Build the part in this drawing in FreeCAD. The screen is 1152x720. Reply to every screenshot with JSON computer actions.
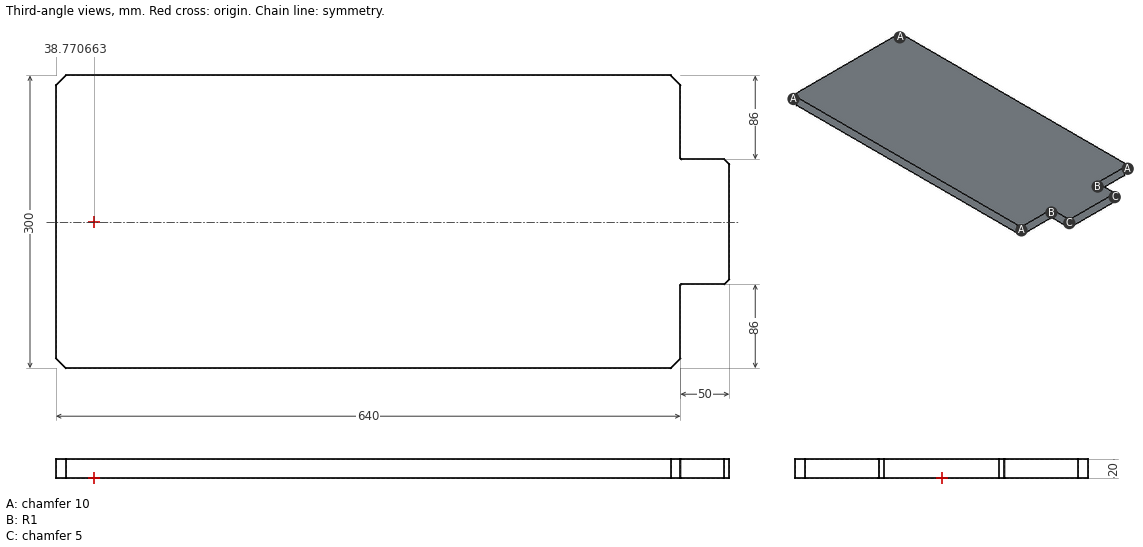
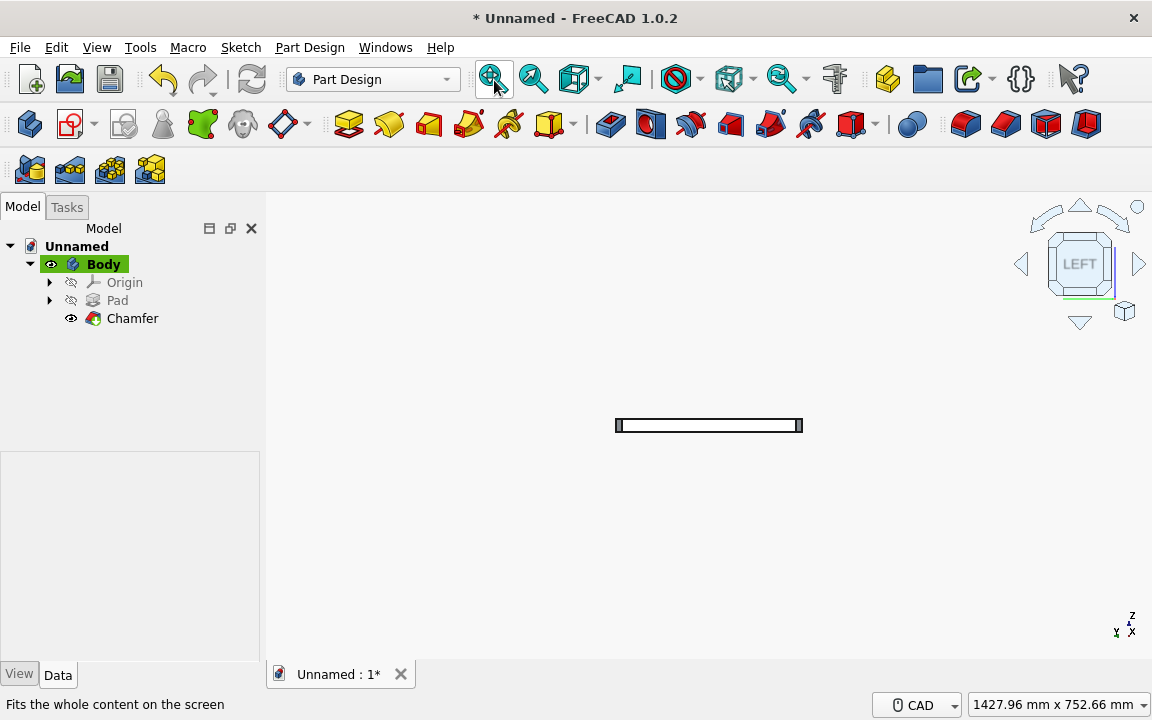
{"action": "left_click", "coordinate": [494, 80]}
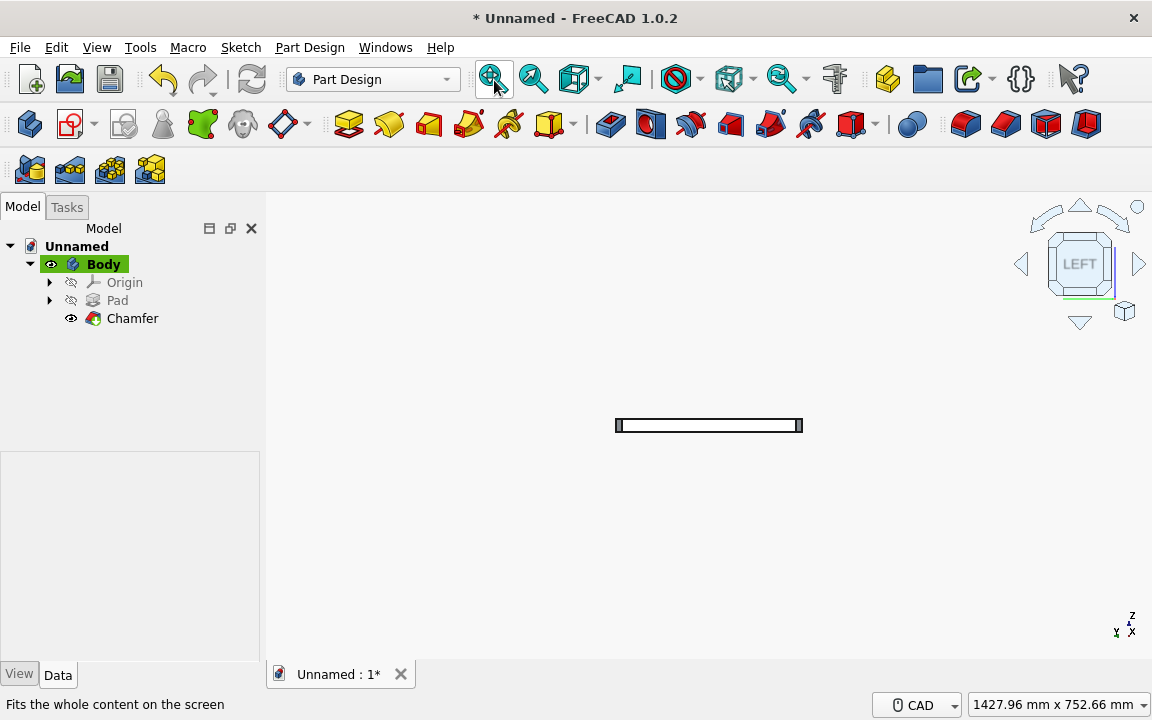
{"action": "scroll", "coordinate": [669, 424], "scroll_direction": "up", "scroll_amount": 6}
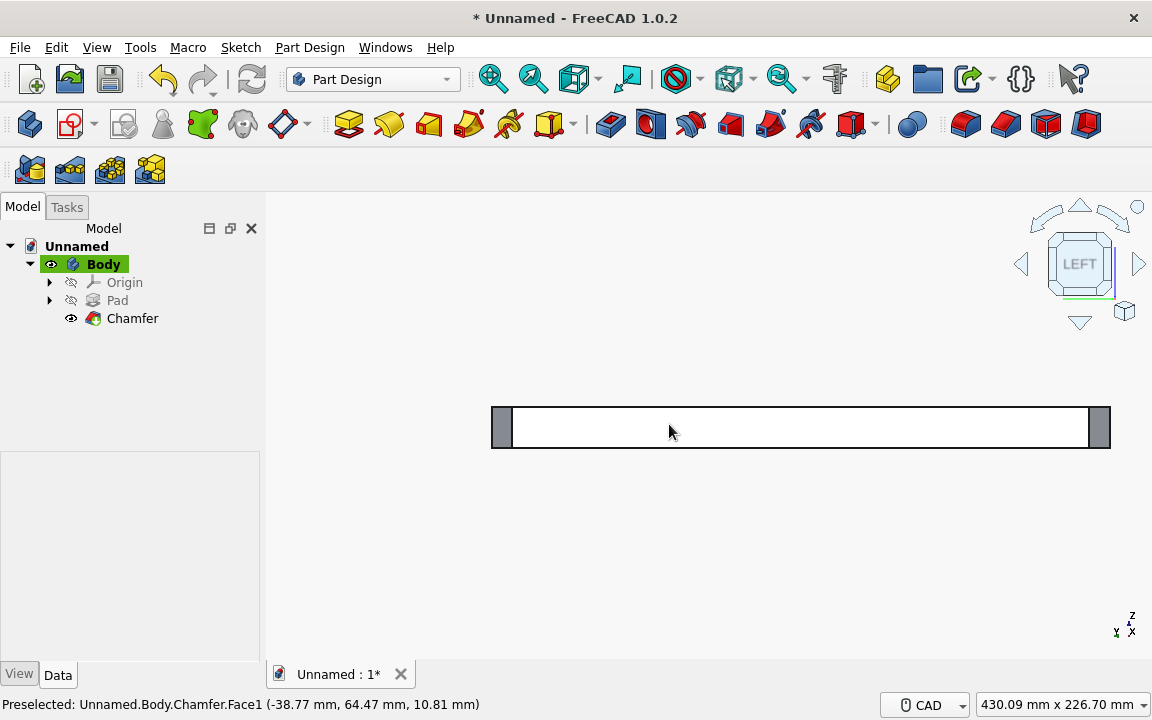
{"action": "key", "text": "v f"}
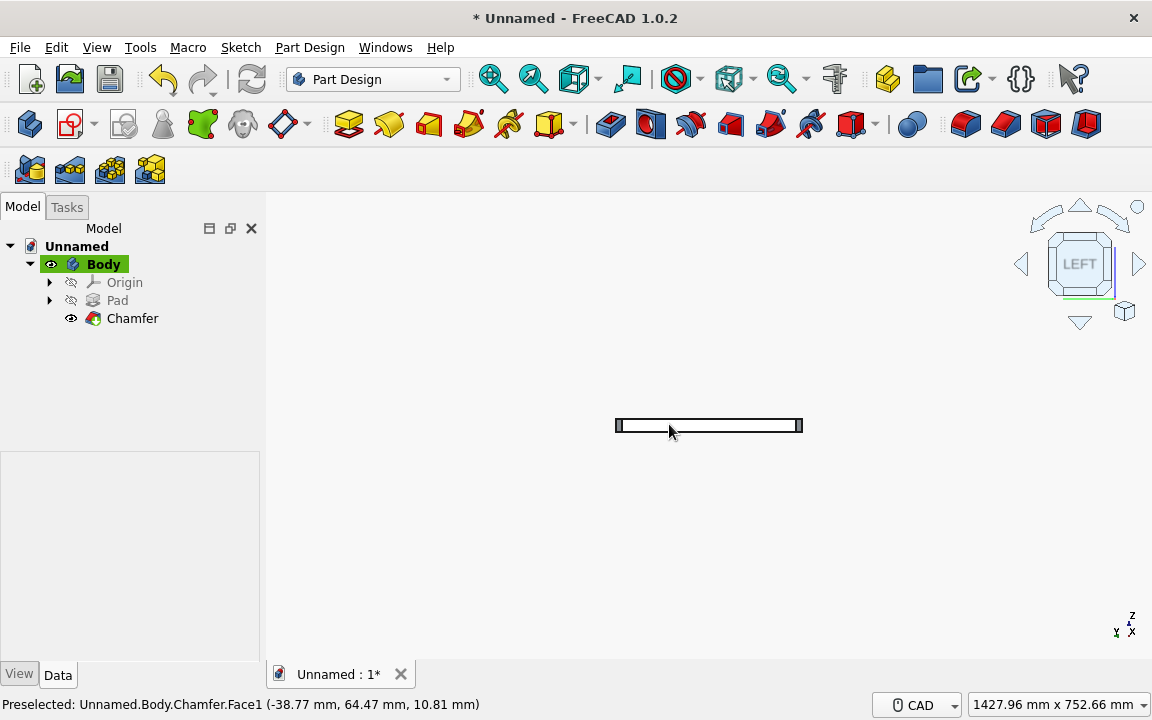
{"action": "key", "text": "v 3"}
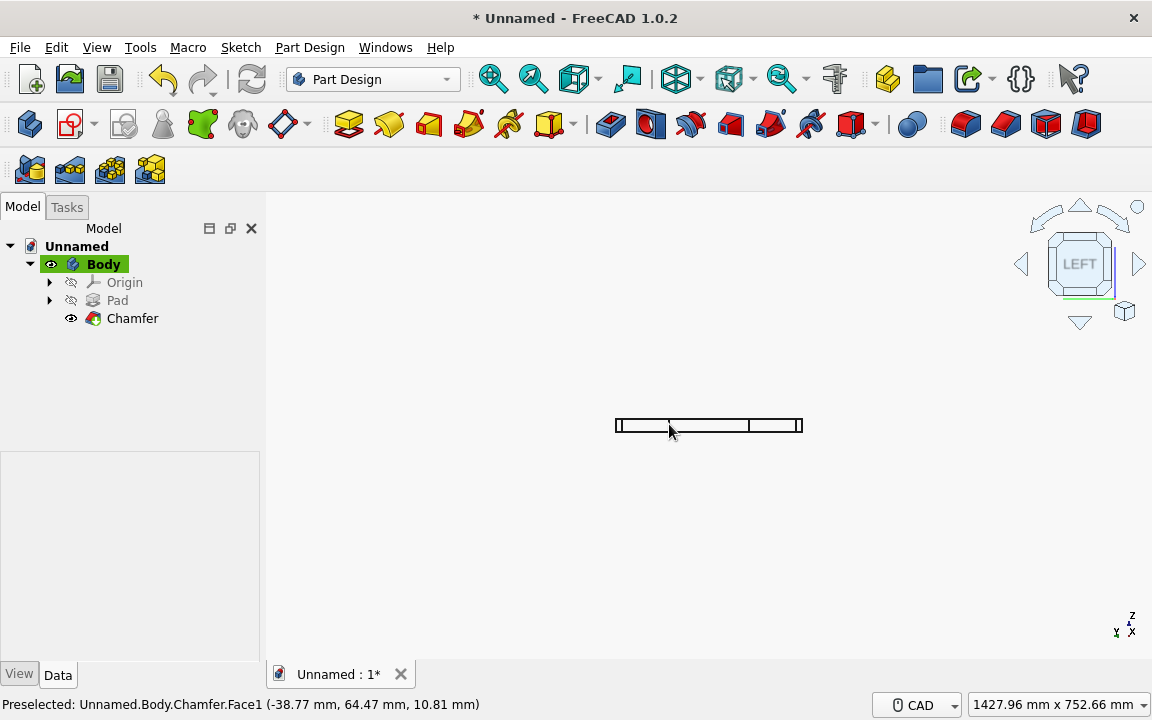
{"action": "key", "text": "0"}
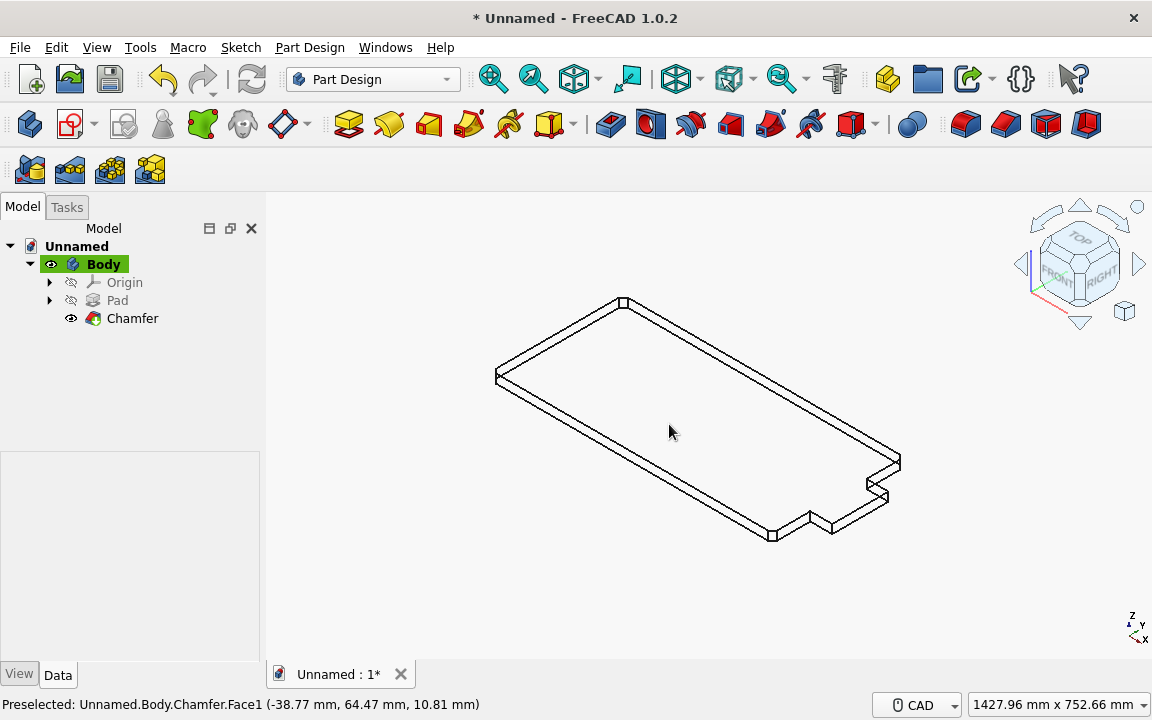
{"action": "left_click", "coordinate": [867, 486]}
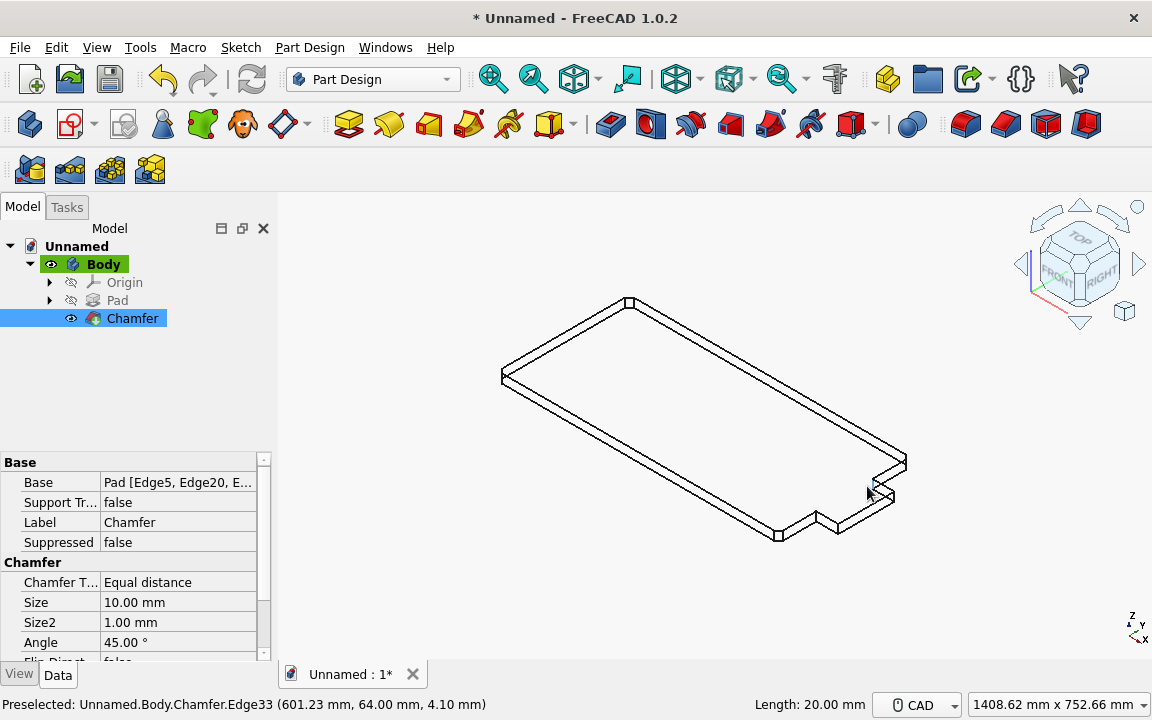
{"action": "left_click", "coordinate": [816, 518], "text": "ctrl"}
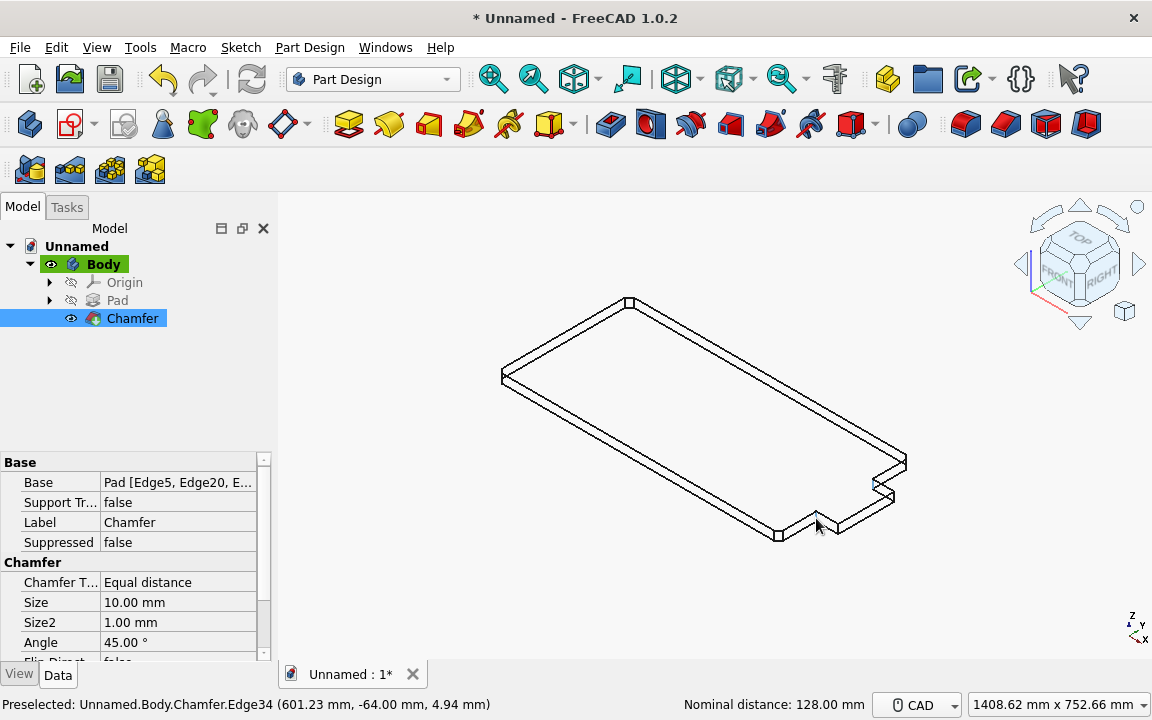
{"action": "key", "text": "v 1"}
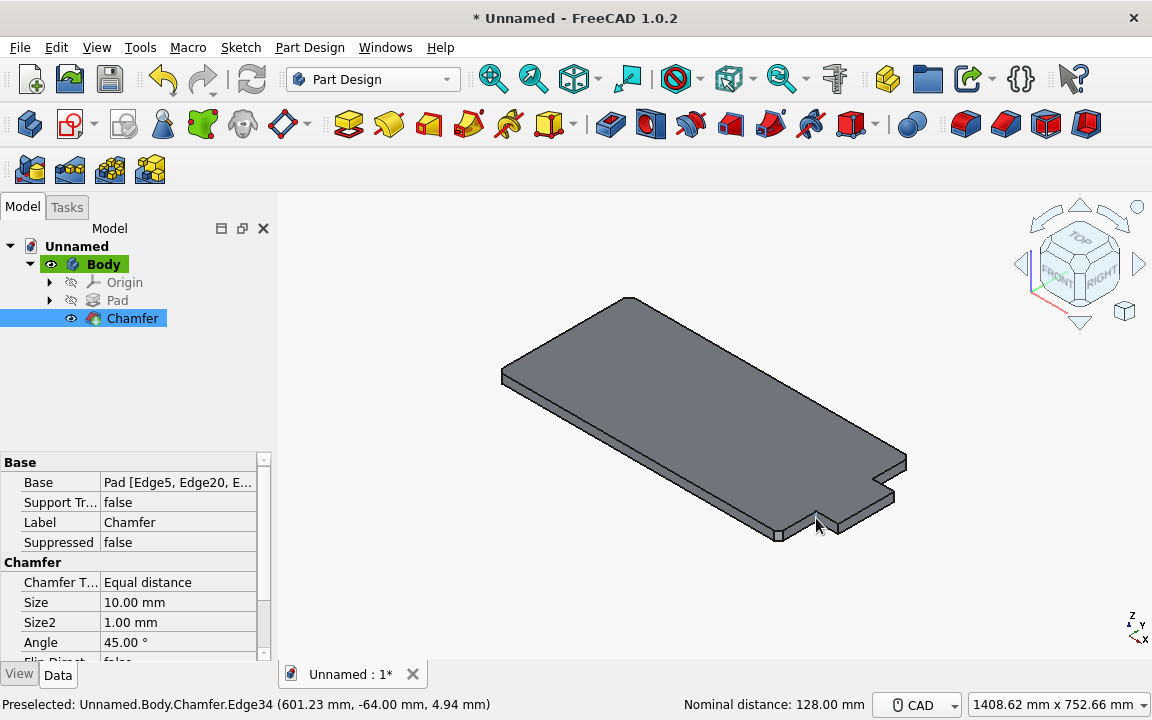
{"action": "left_click", "coordinate": [966, 124]}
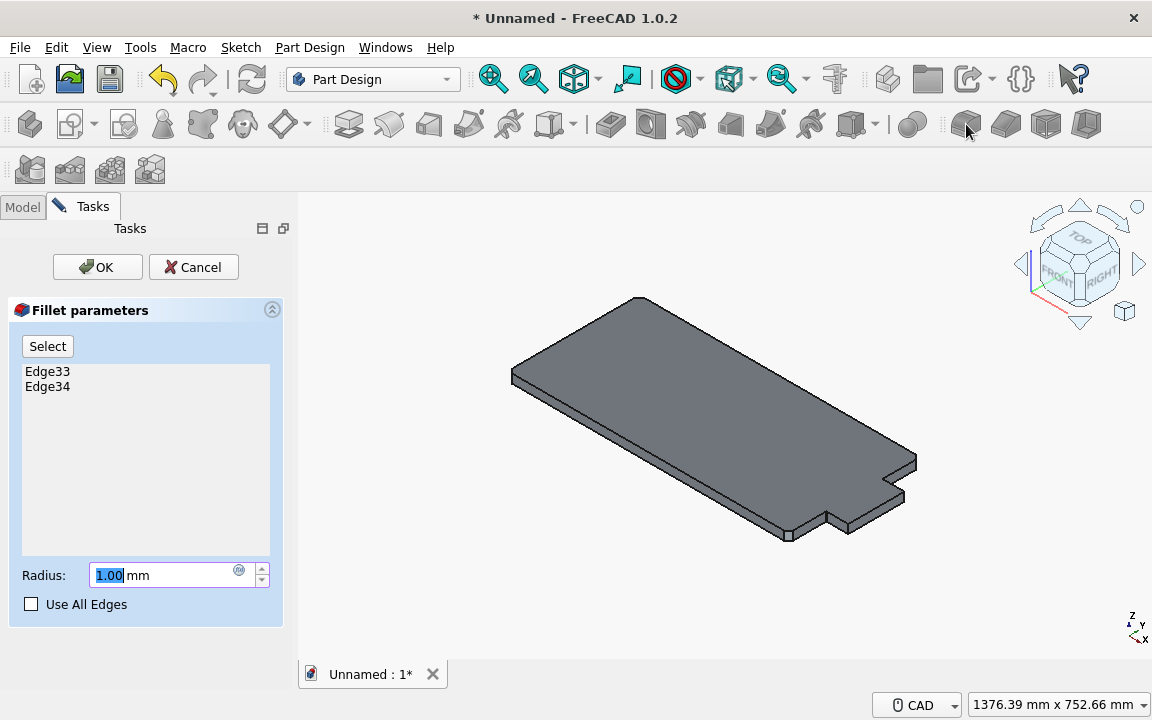
{"action": "type", "text": "1"}
{"action": "key", "text": "Tab"}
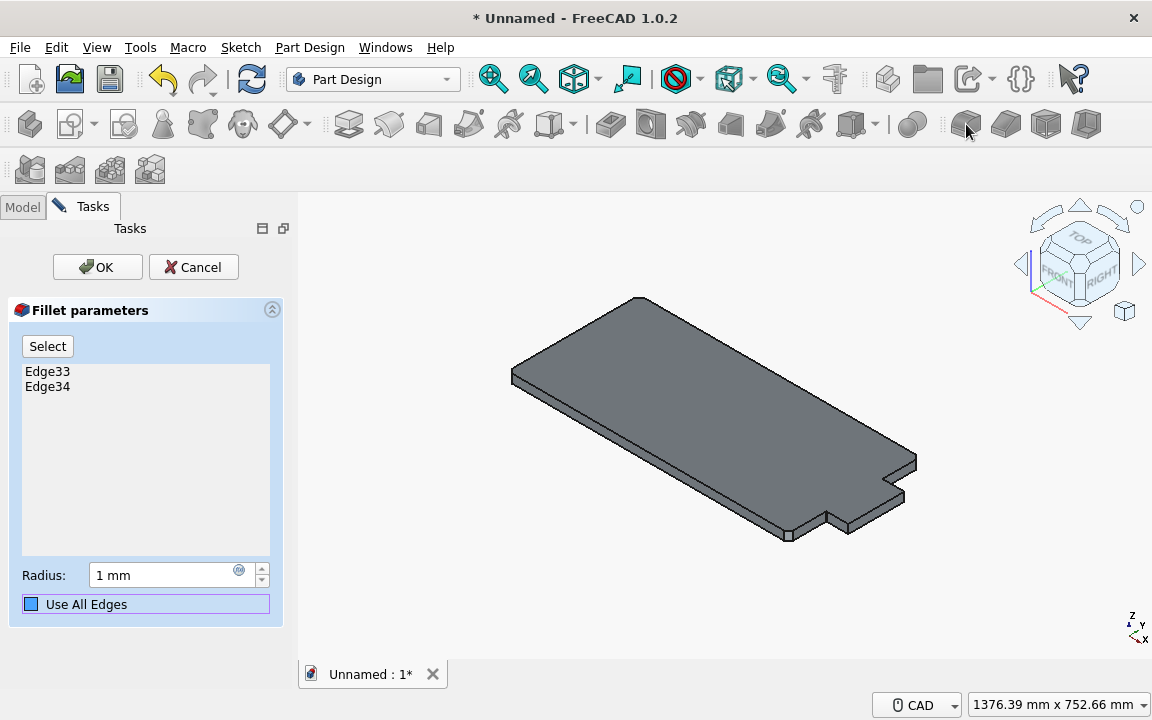
{"action": "left_click", "coordinate": [98, 267]}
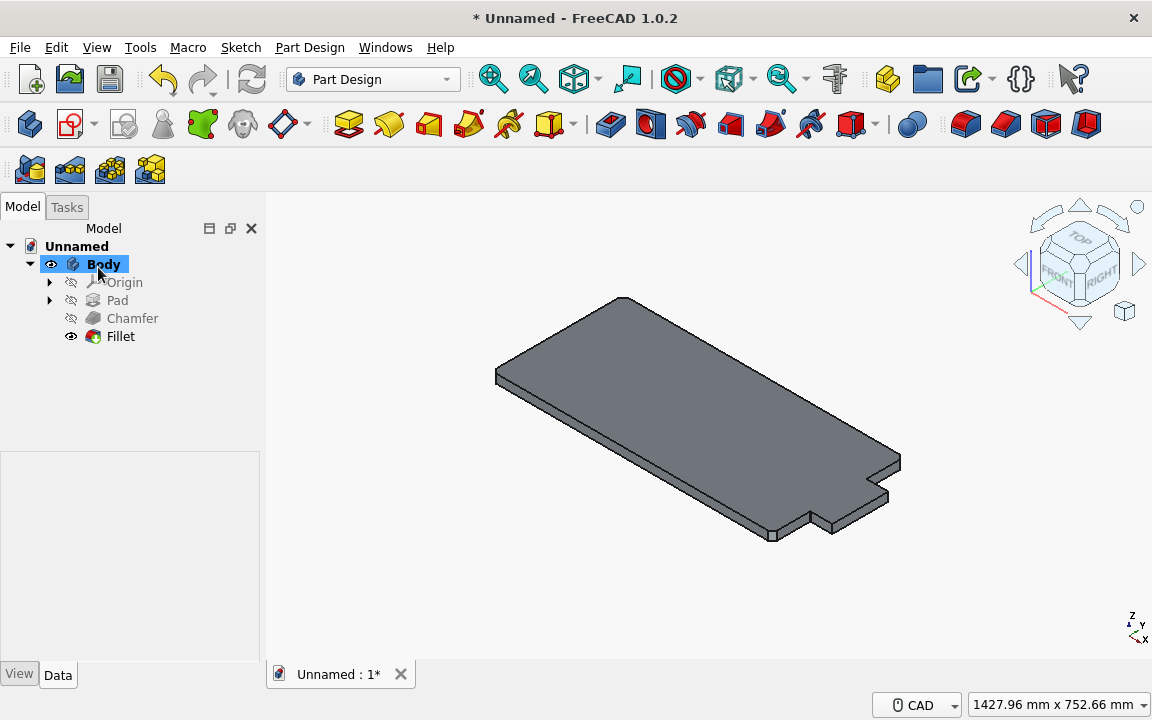
{"action": "left_click", "coordinate": [832, 529]}